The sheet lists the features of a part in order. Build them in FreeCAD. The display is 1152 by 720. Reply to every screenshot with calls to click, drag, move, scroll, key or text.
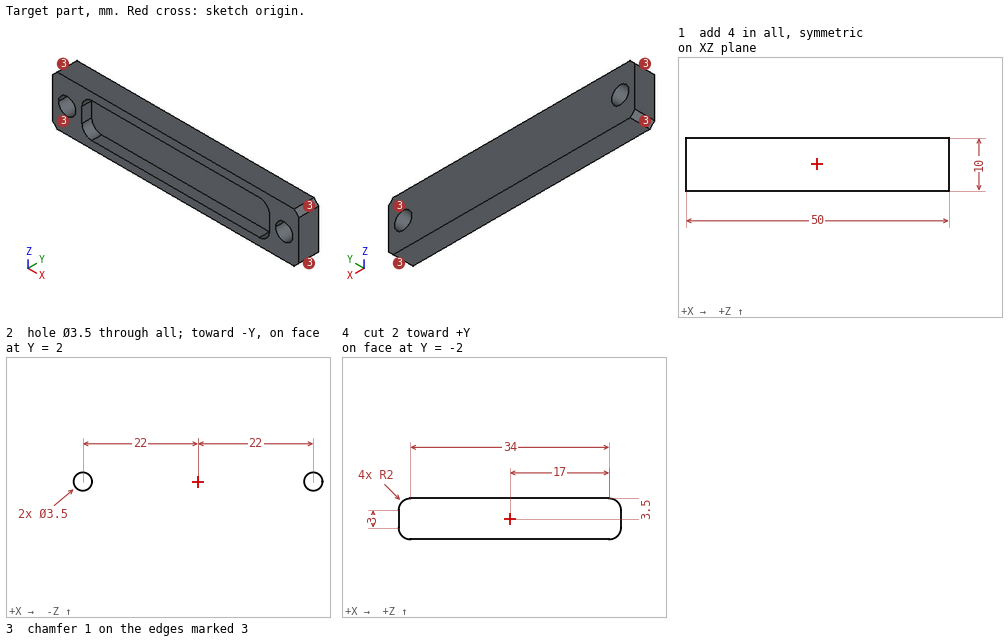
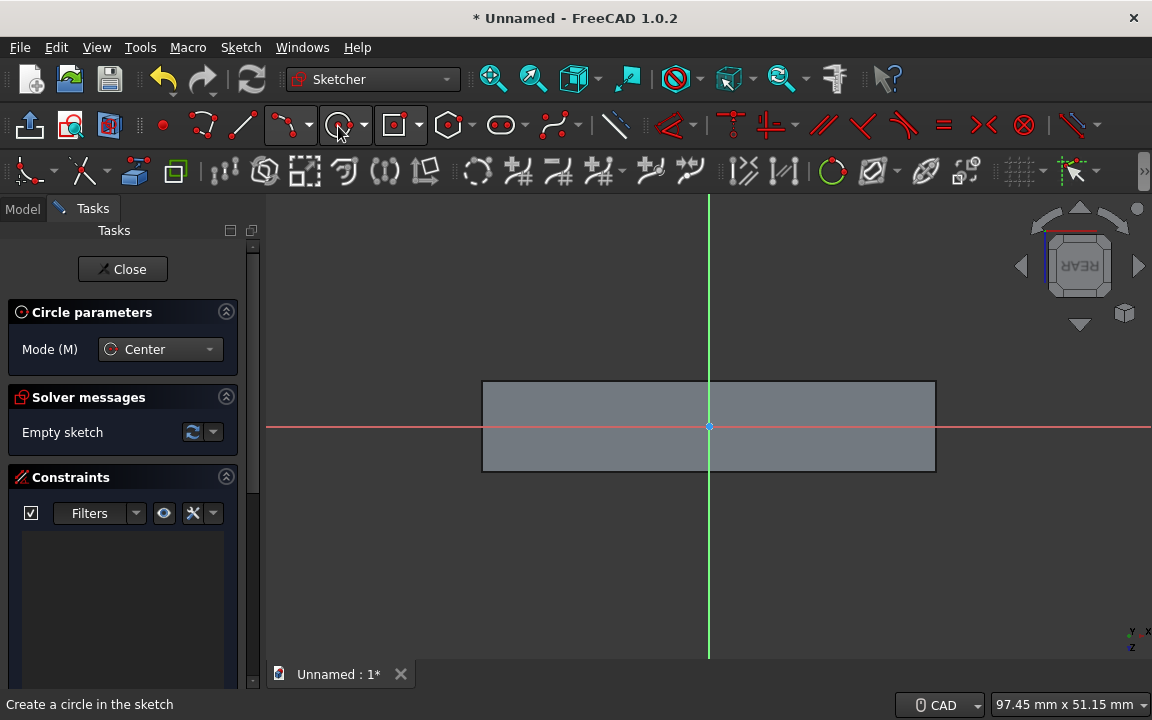
scroll(509, 427, up, 2)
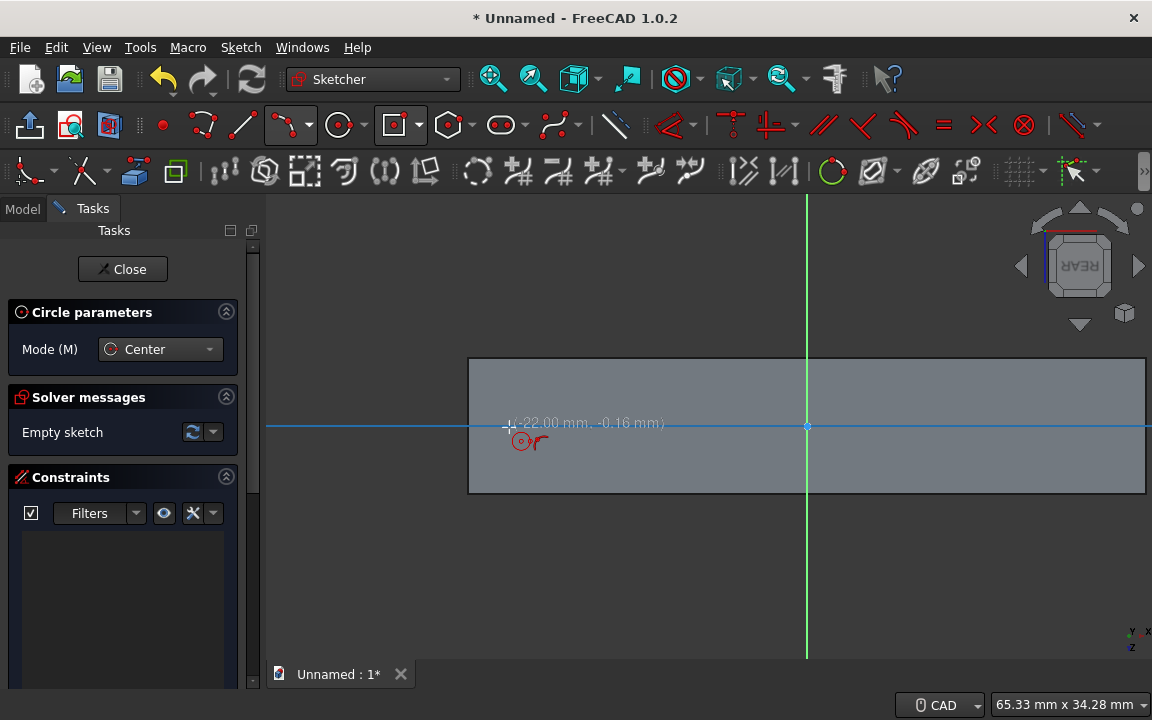
click(509, 426)
click(526, 409)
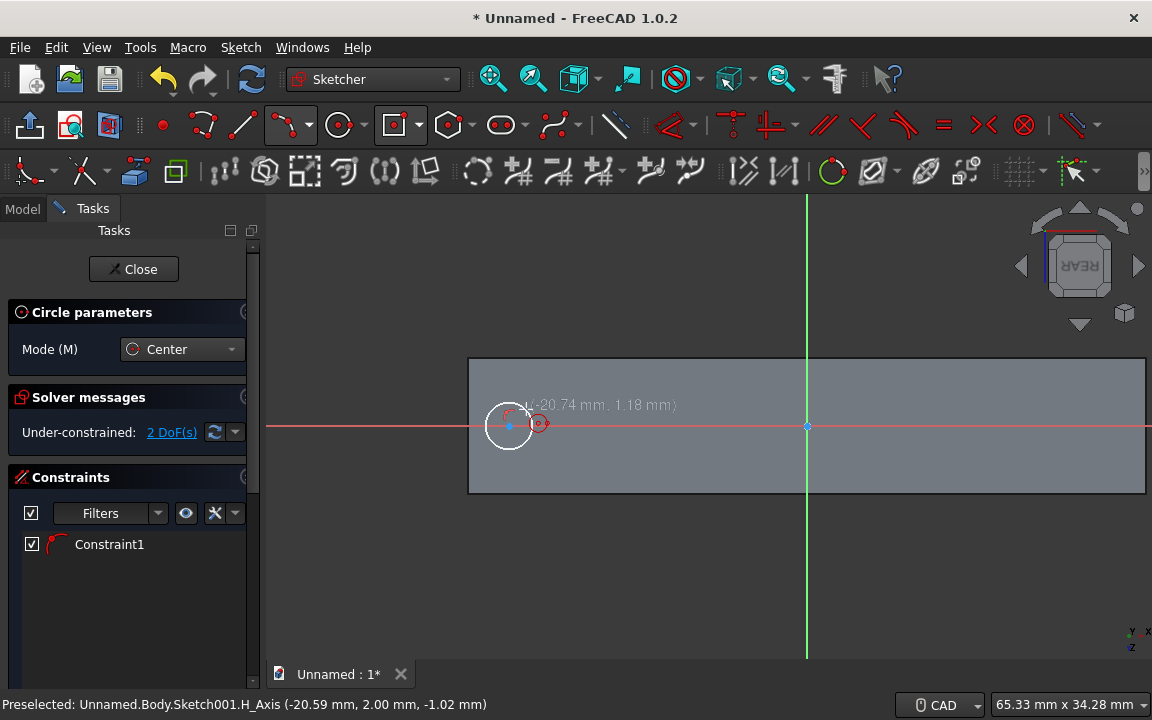
scroll(301, 428, down, 2)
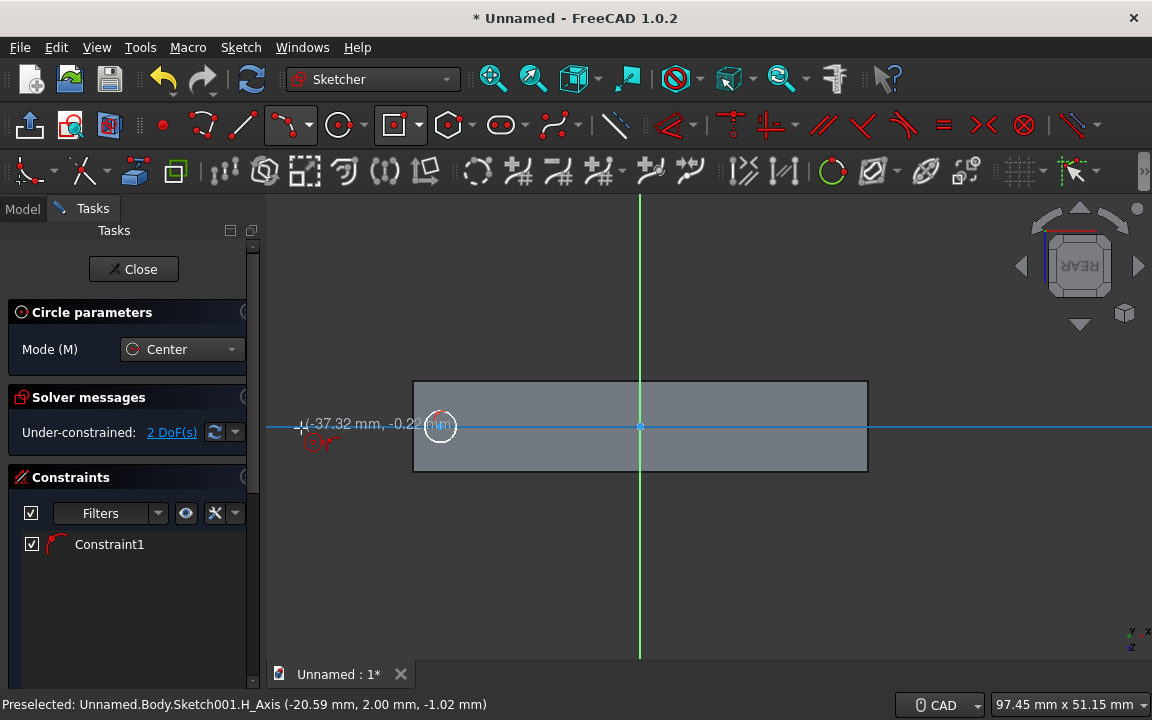
scroll(840, 427, up, 2)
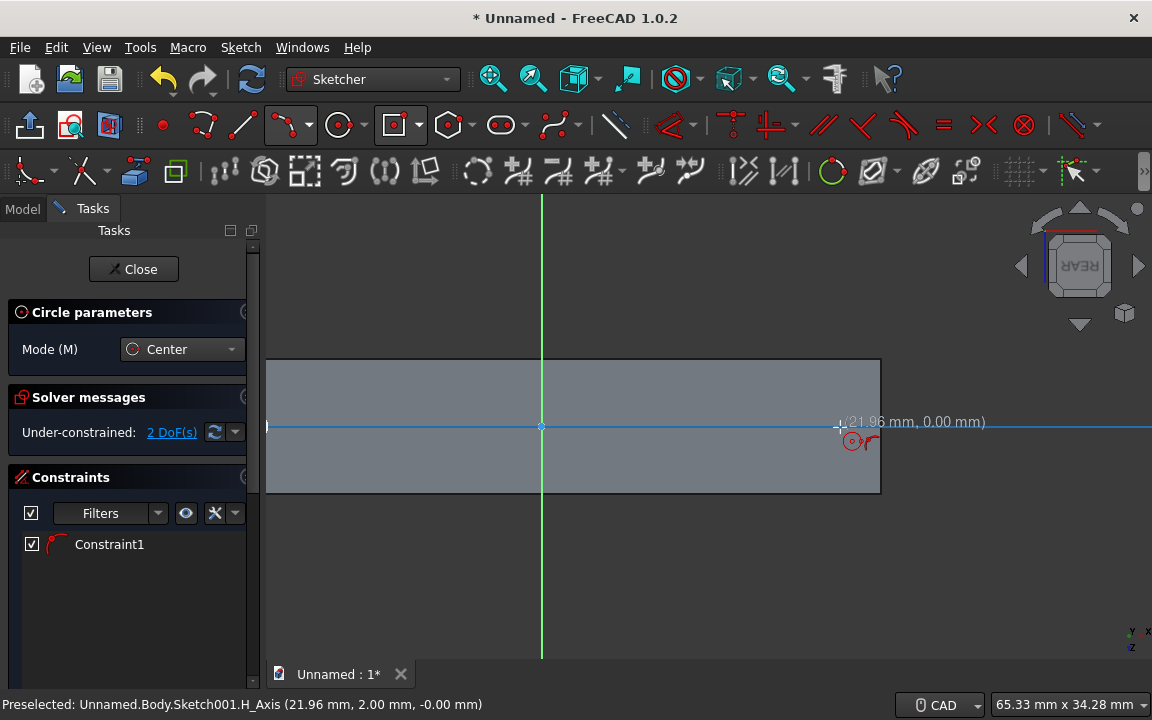
click(840, 427)
click(857, 410)
key(Escape)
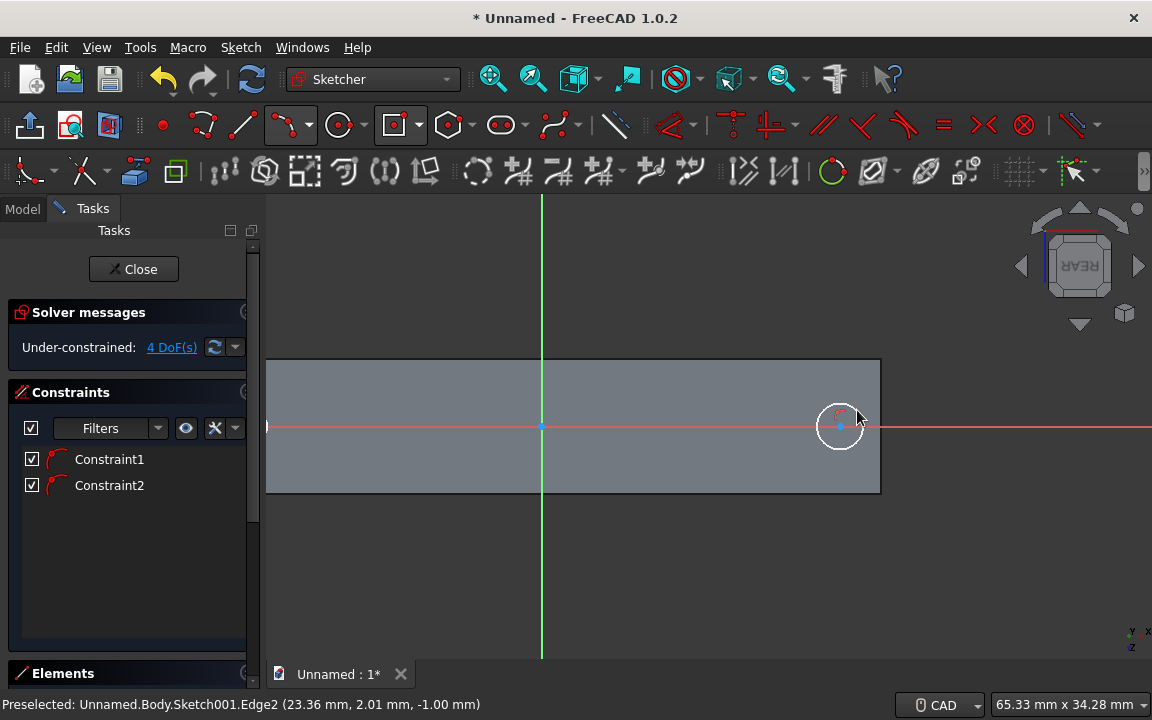
scroll(987, 426, down, 1)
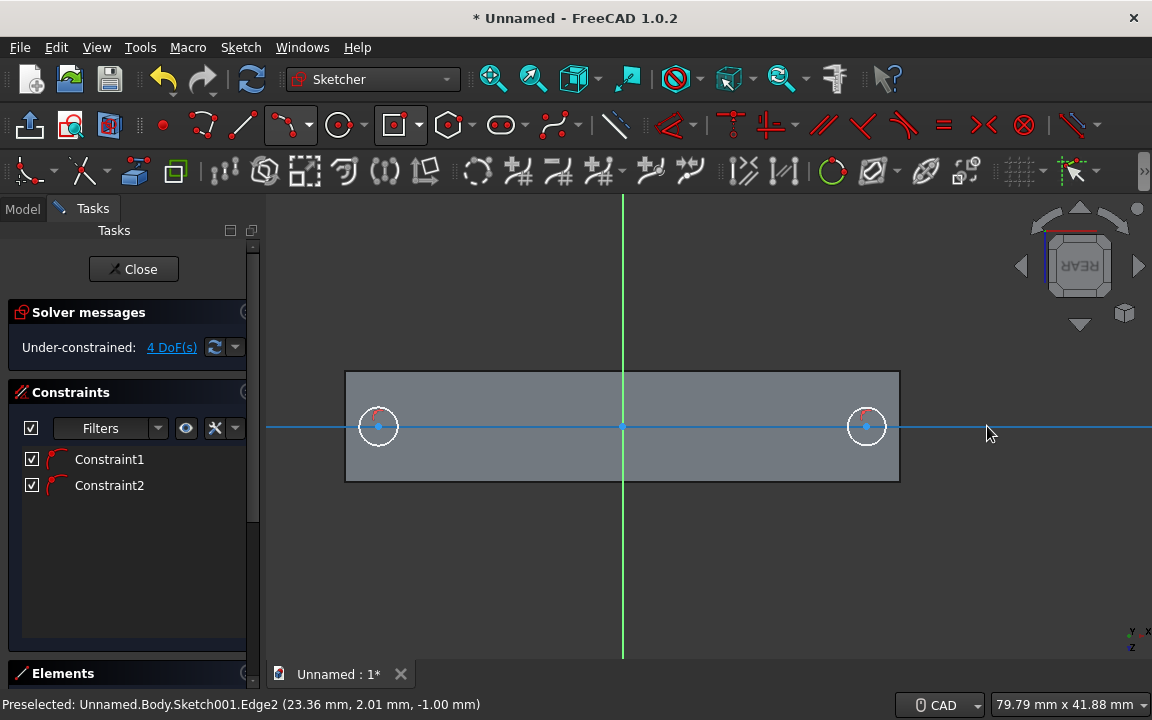
click(392, 413)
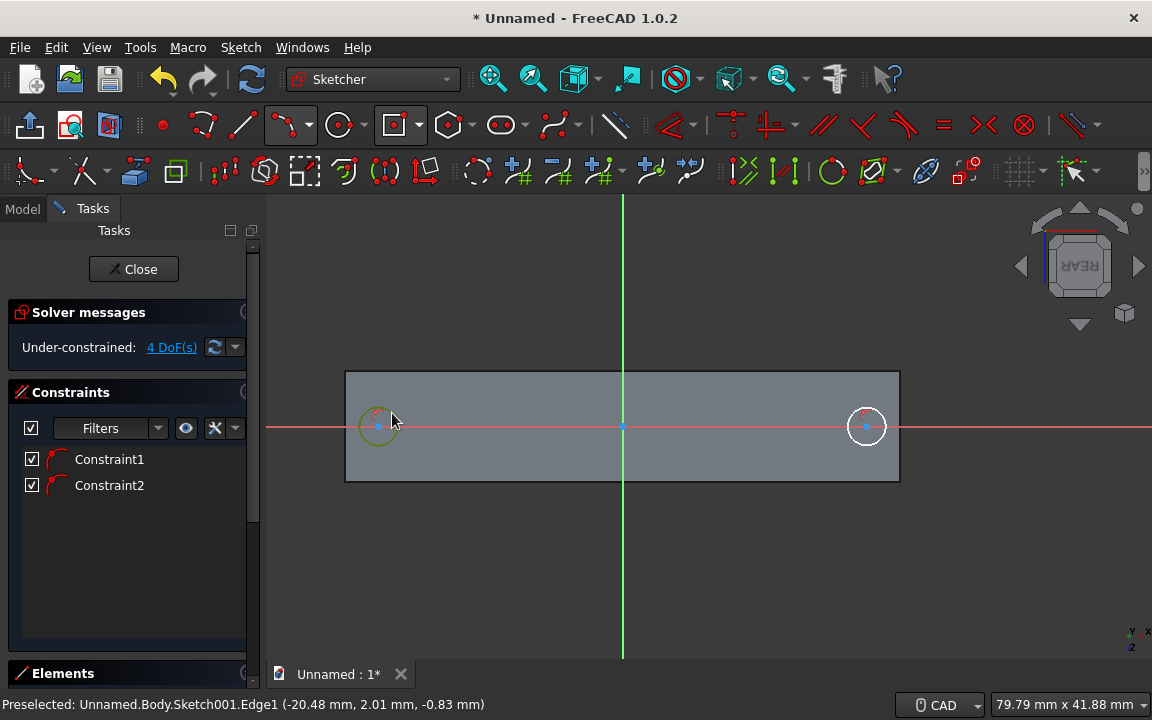
click(880, 413)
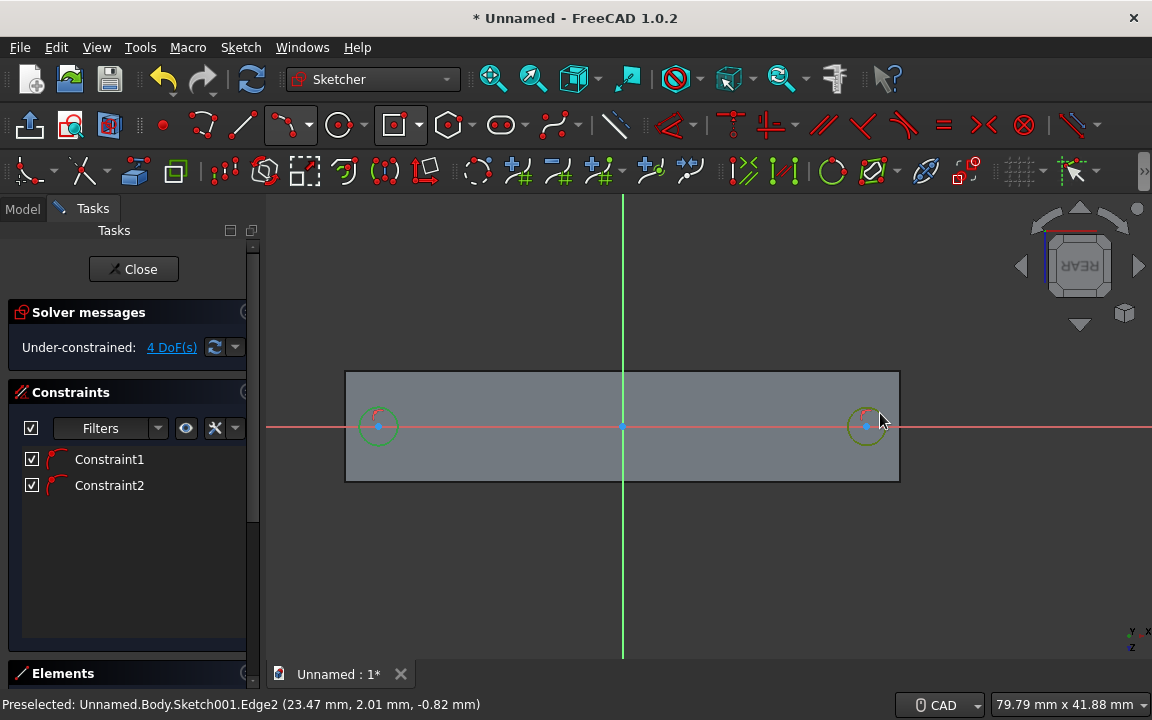
click(944, 126)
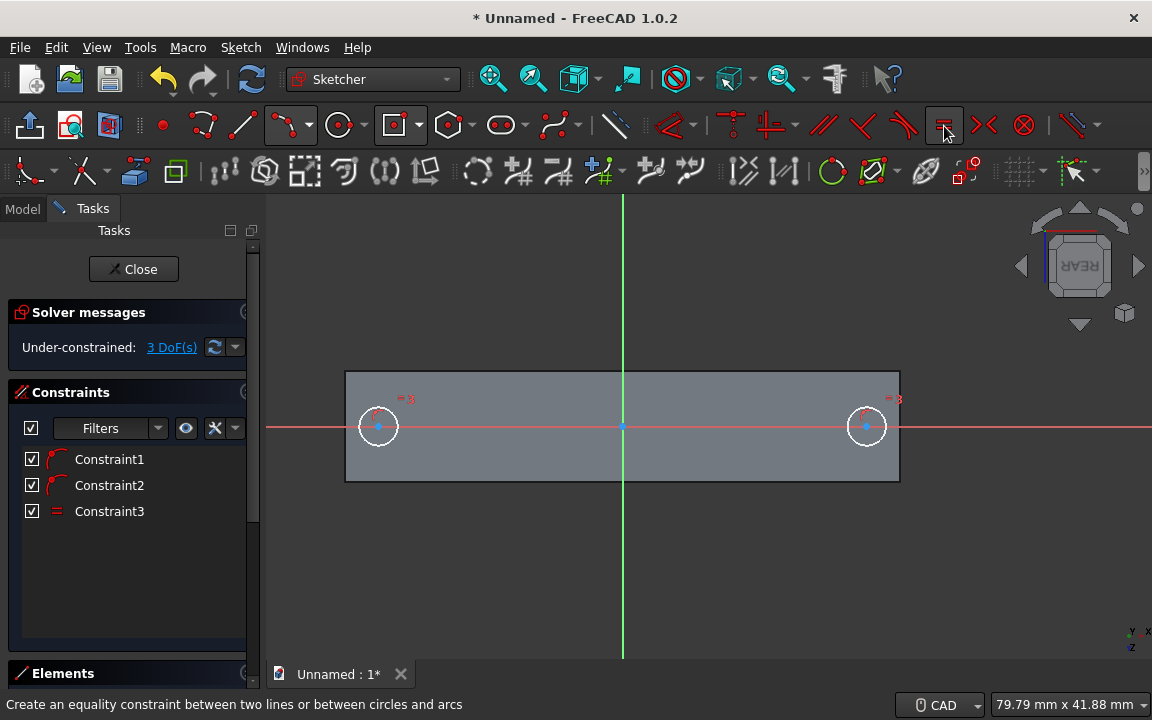
click(392, 413)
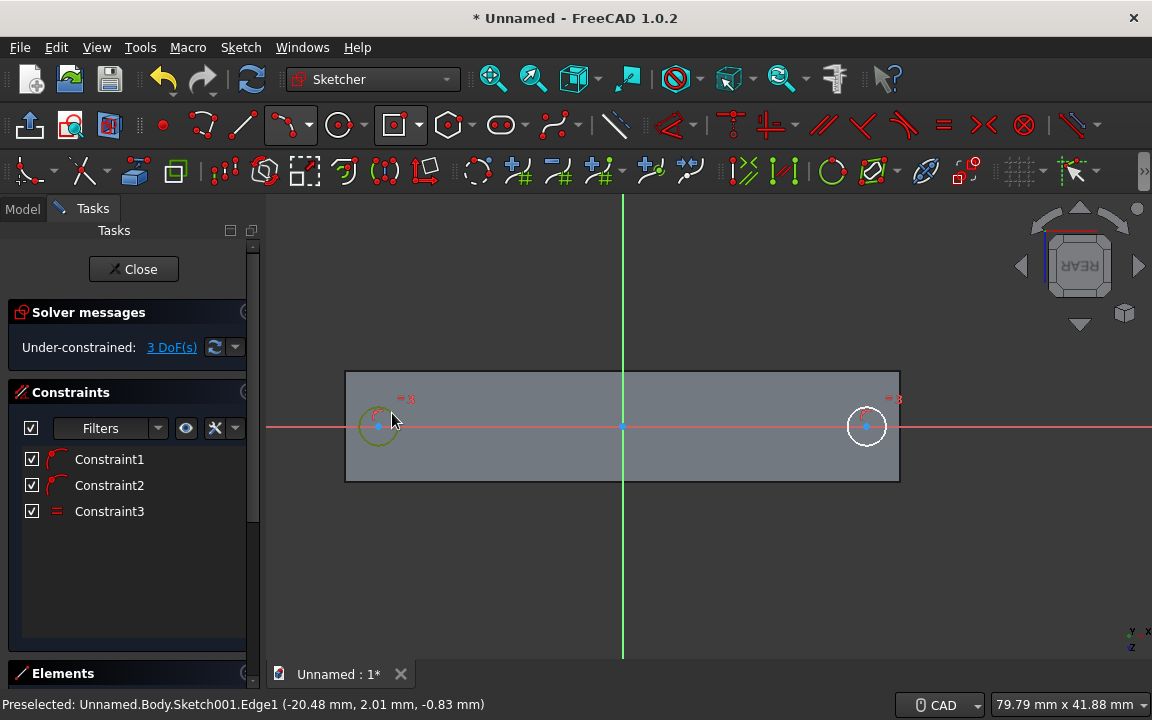
click(696, 126)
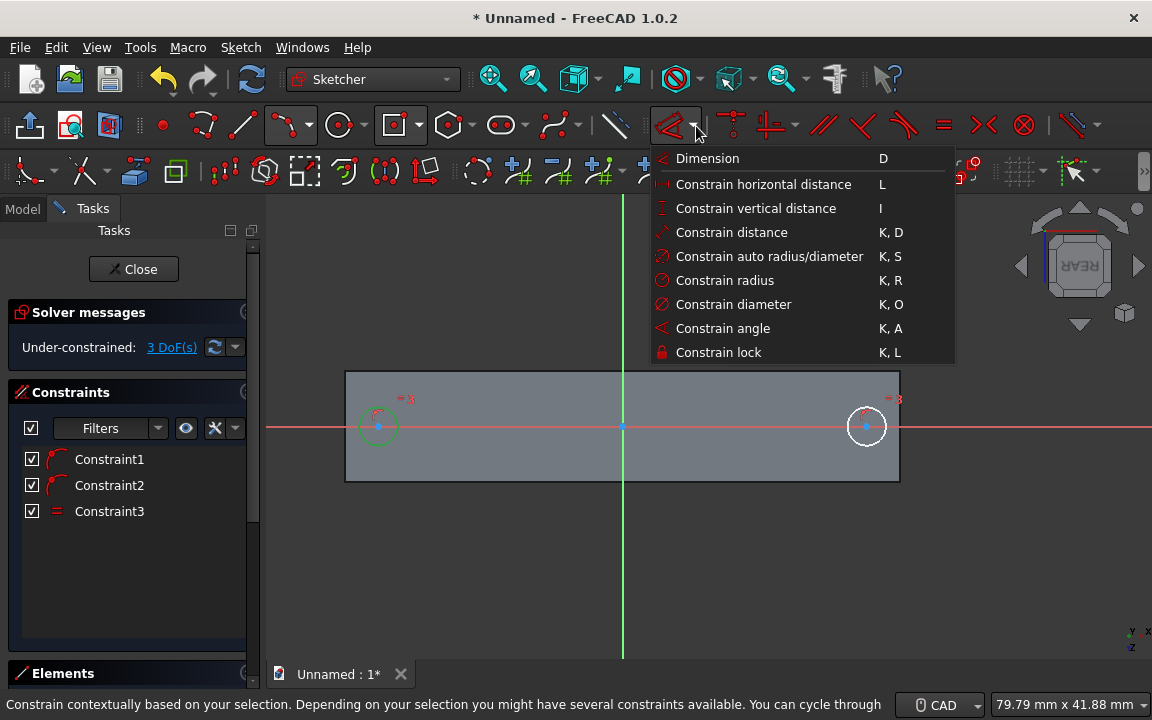
click(803, 304)